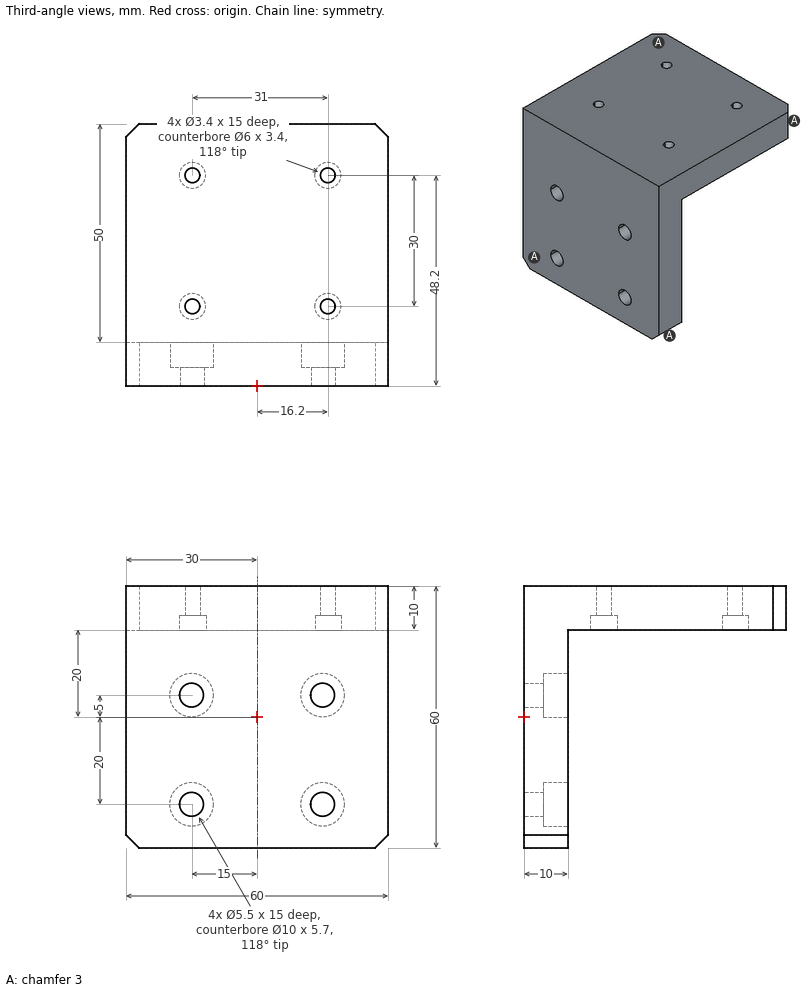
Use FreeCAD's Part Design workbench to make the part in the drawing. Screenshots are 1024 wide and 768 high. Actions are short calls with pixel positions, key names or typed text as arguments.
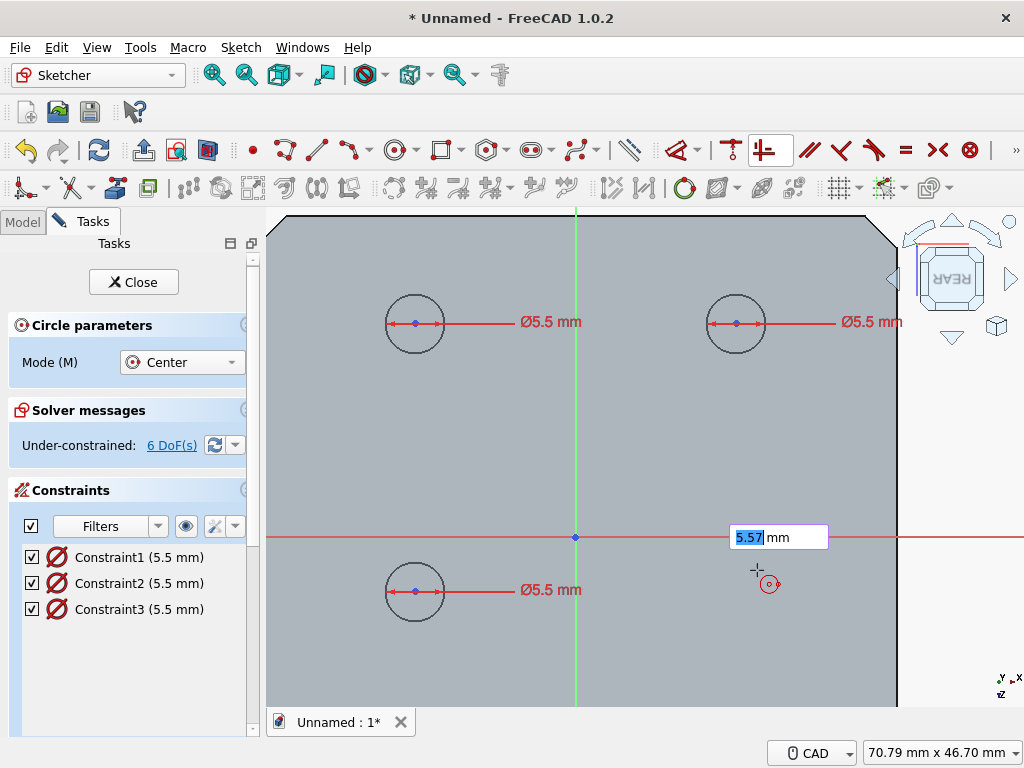
text(5.5)
key(Return)
key(Escape)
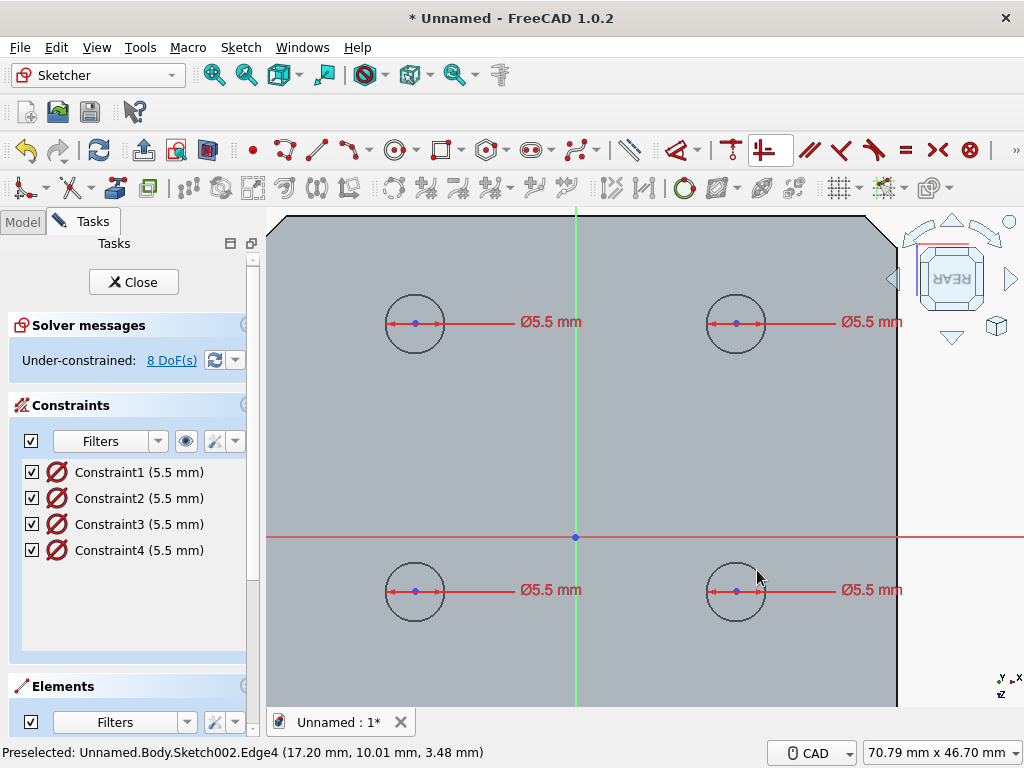
click(415, 324)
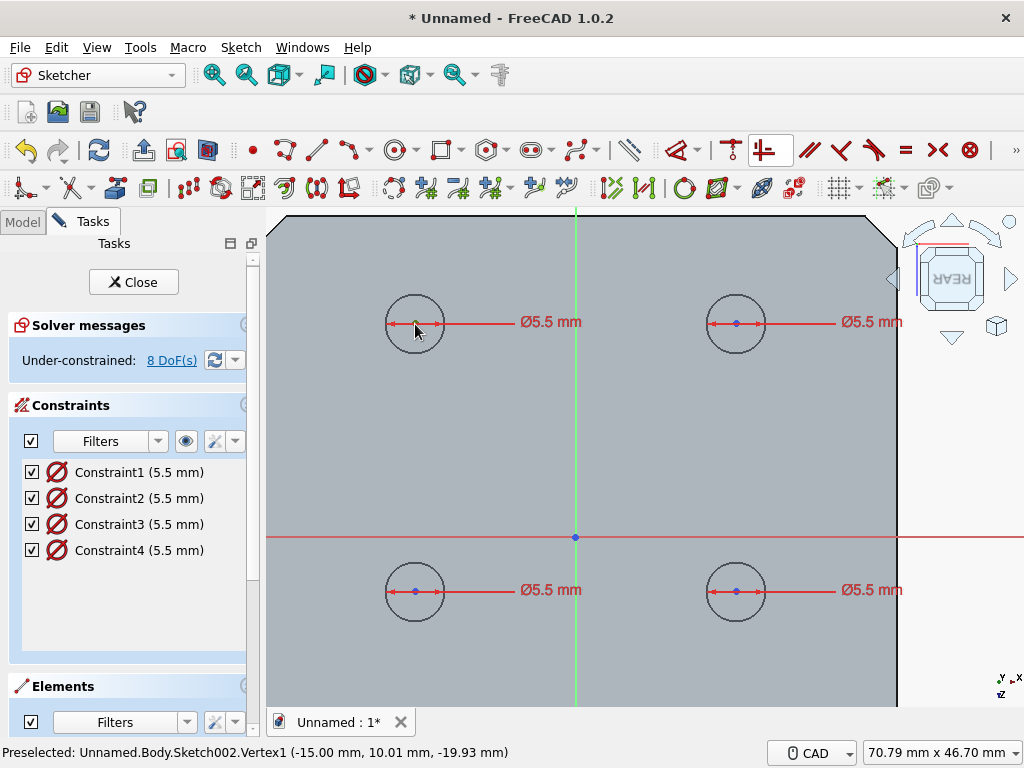
click(736, 324)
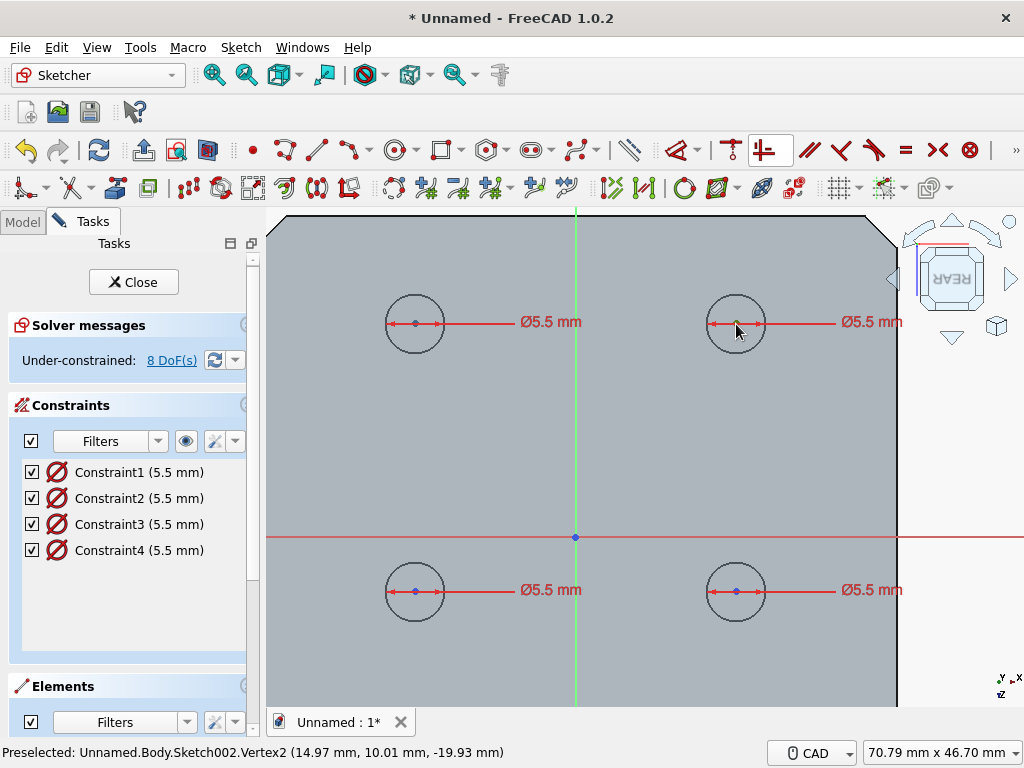
click(576, 647)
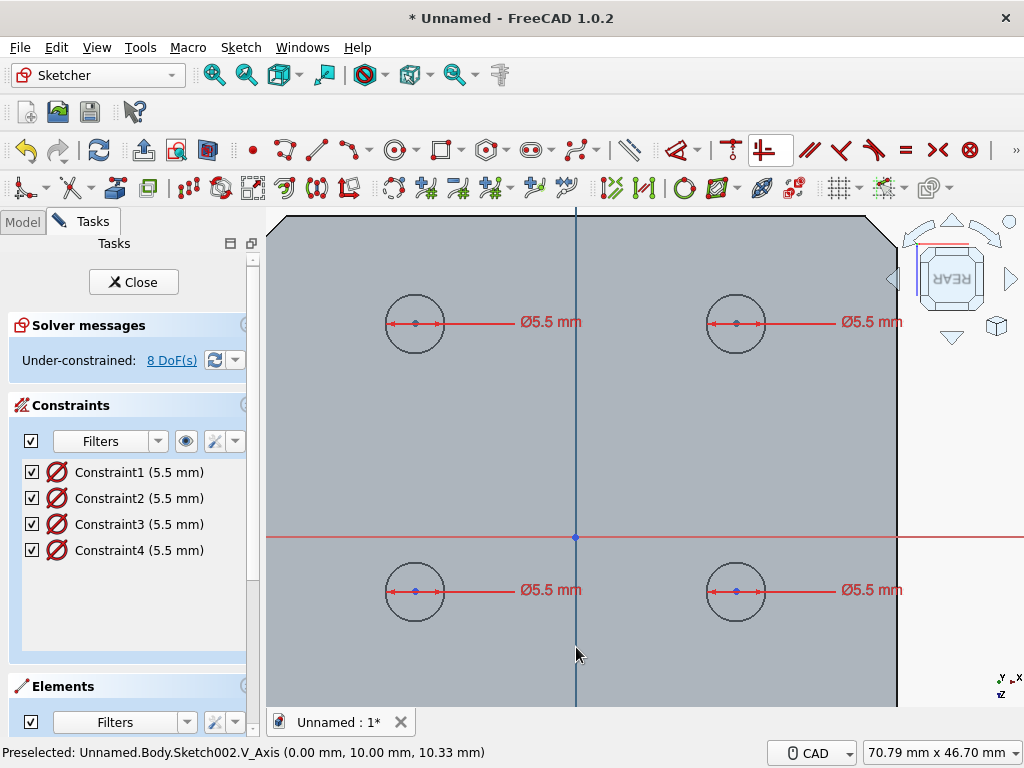
key(s)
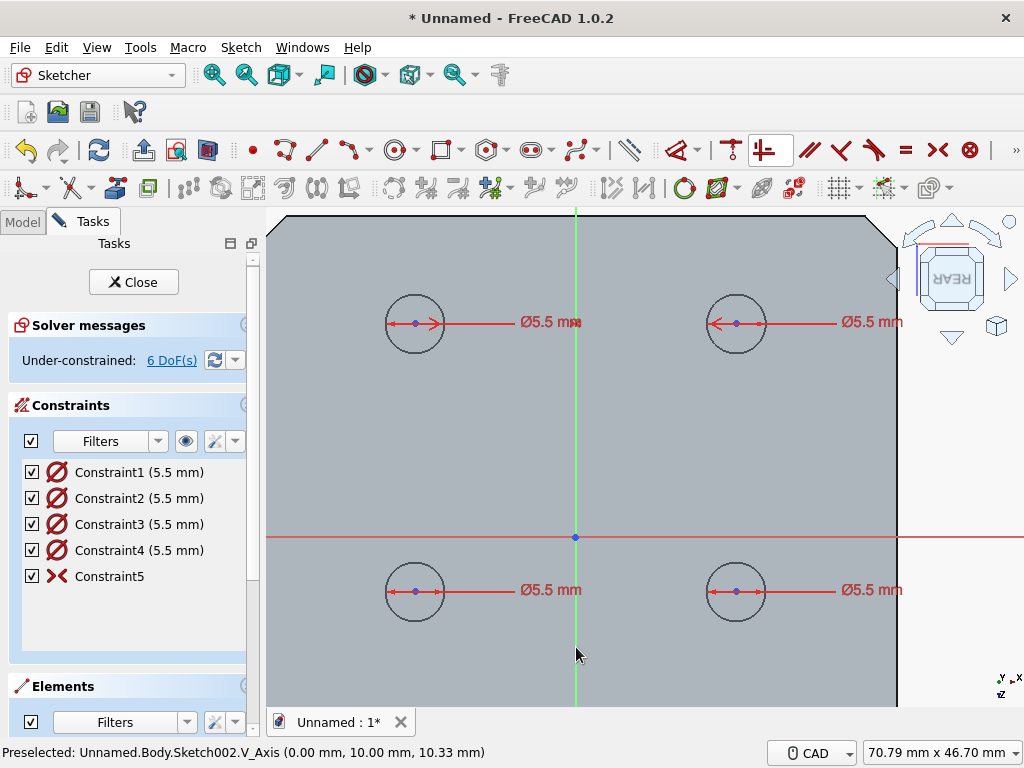
click(415, 592)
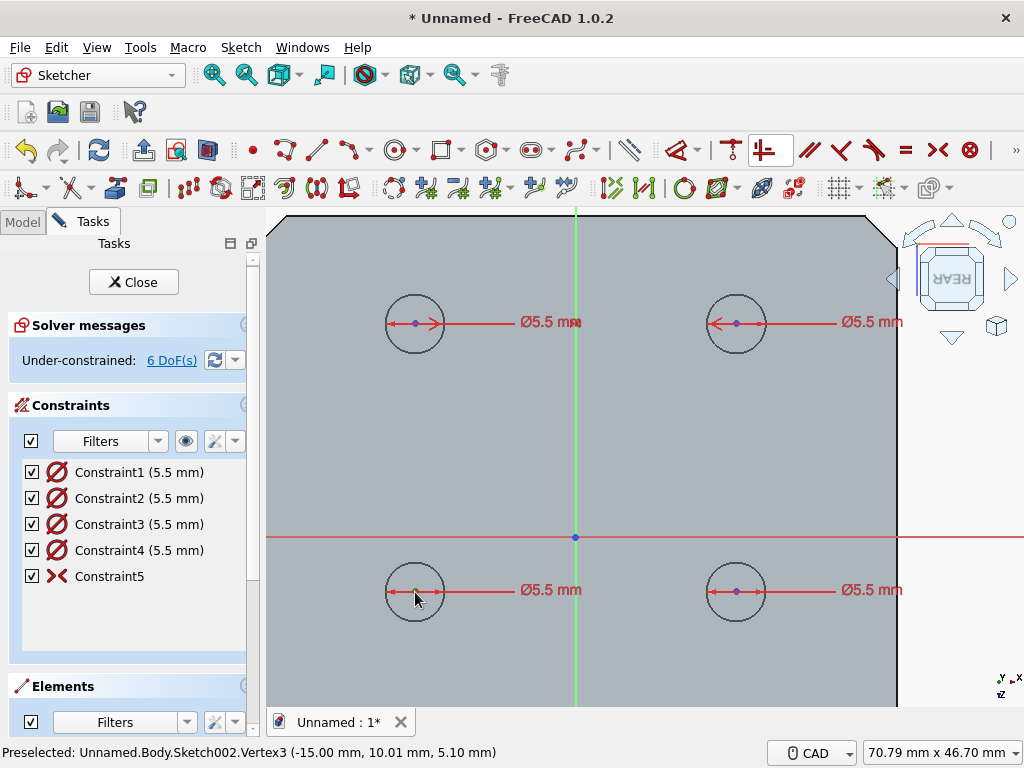
click(736, 592)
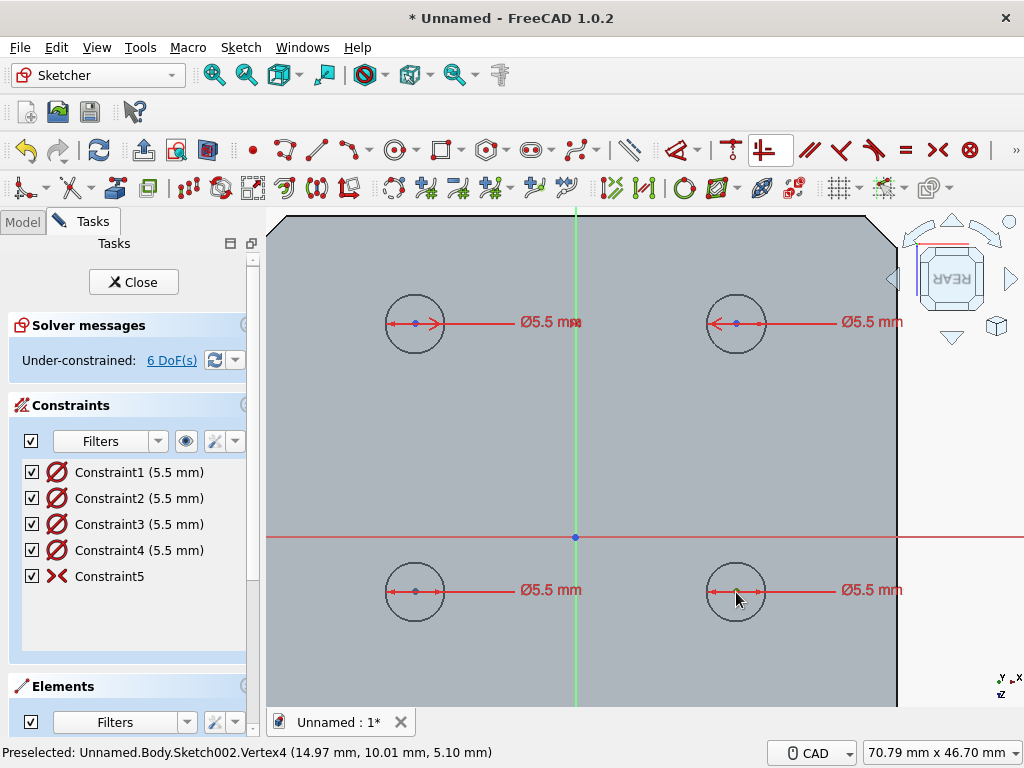
click(576, 647)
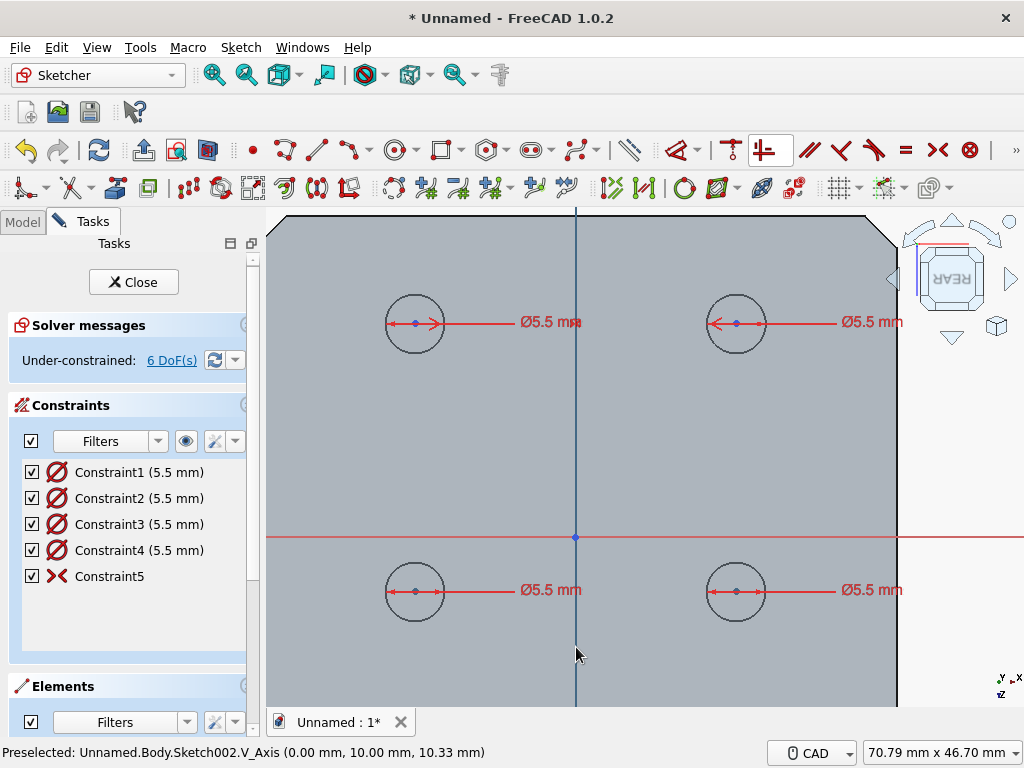
click(938, 150)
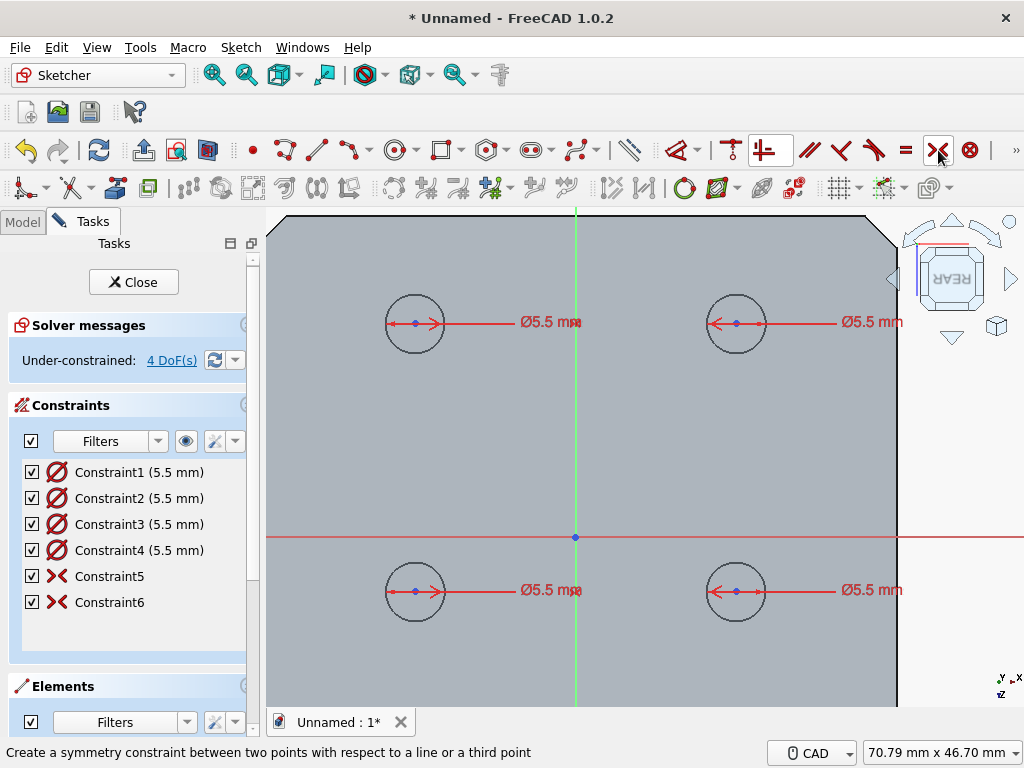
click(676, 150)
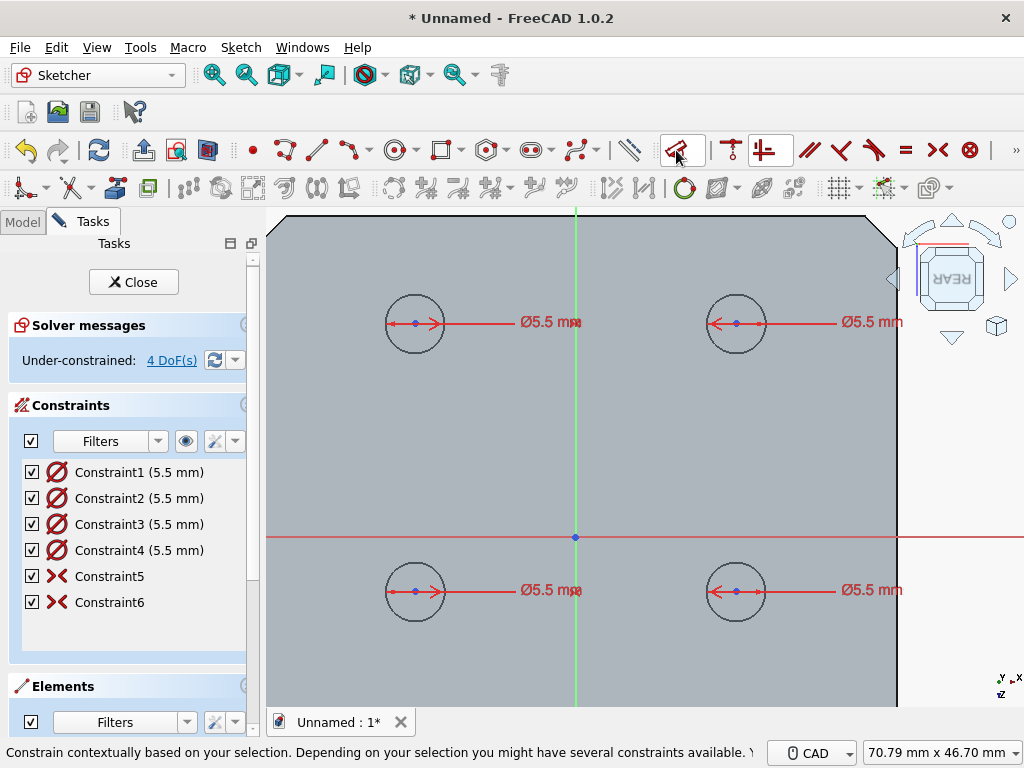
click(415, 592)
click(381, 565)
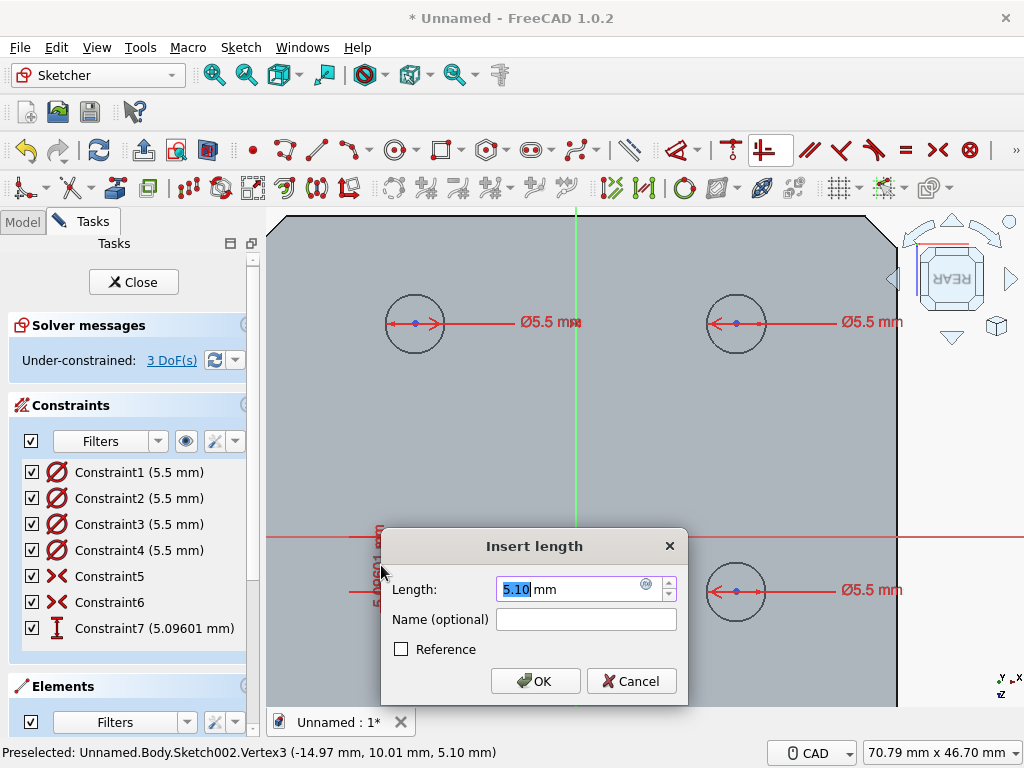
text(5)
key(Return)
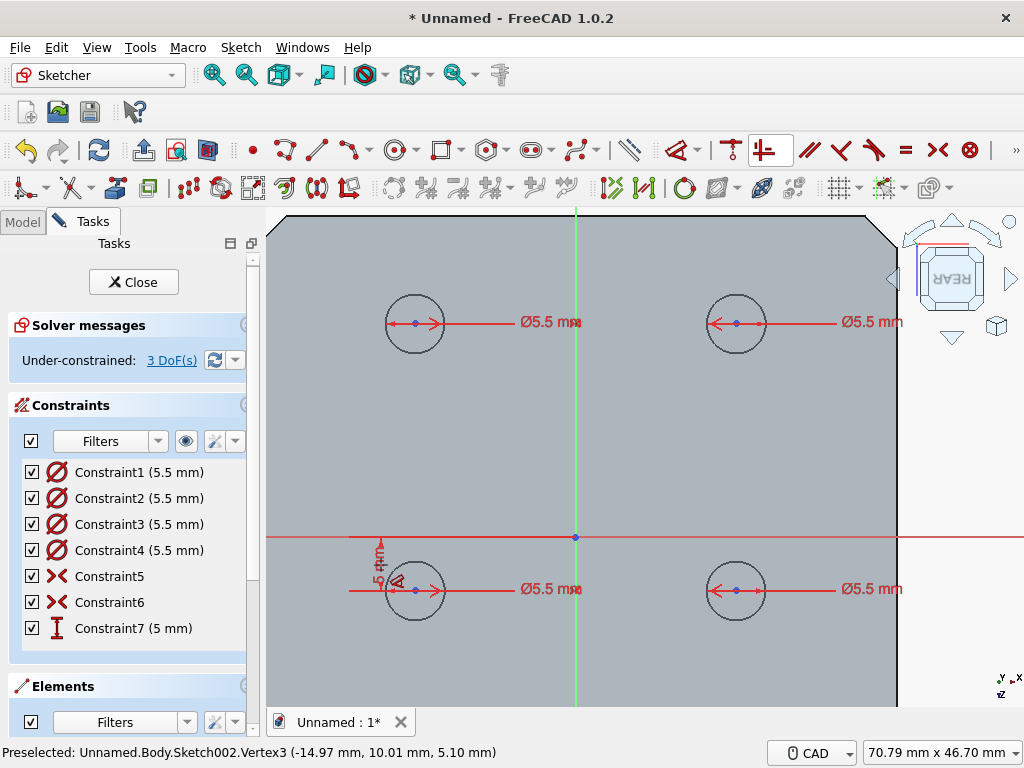
click(415, 324)
click(495, 290)